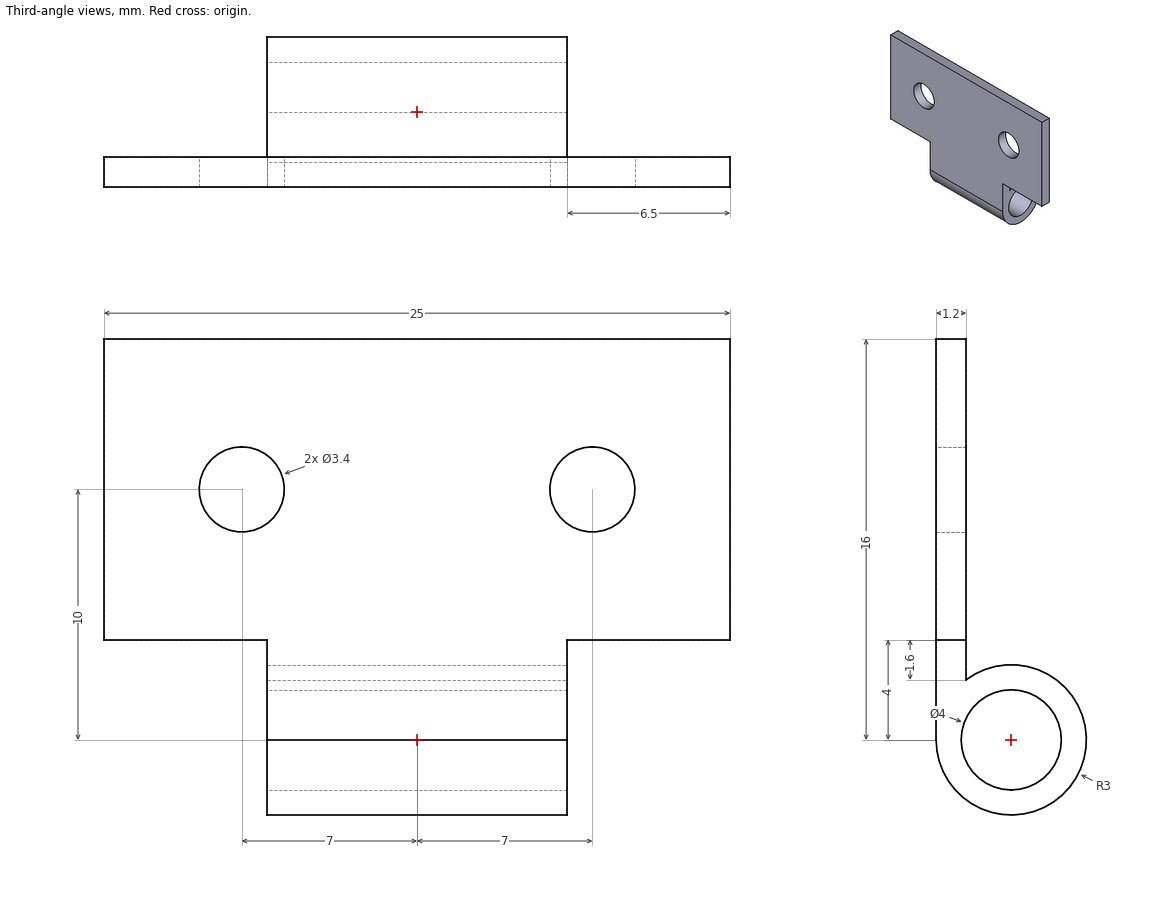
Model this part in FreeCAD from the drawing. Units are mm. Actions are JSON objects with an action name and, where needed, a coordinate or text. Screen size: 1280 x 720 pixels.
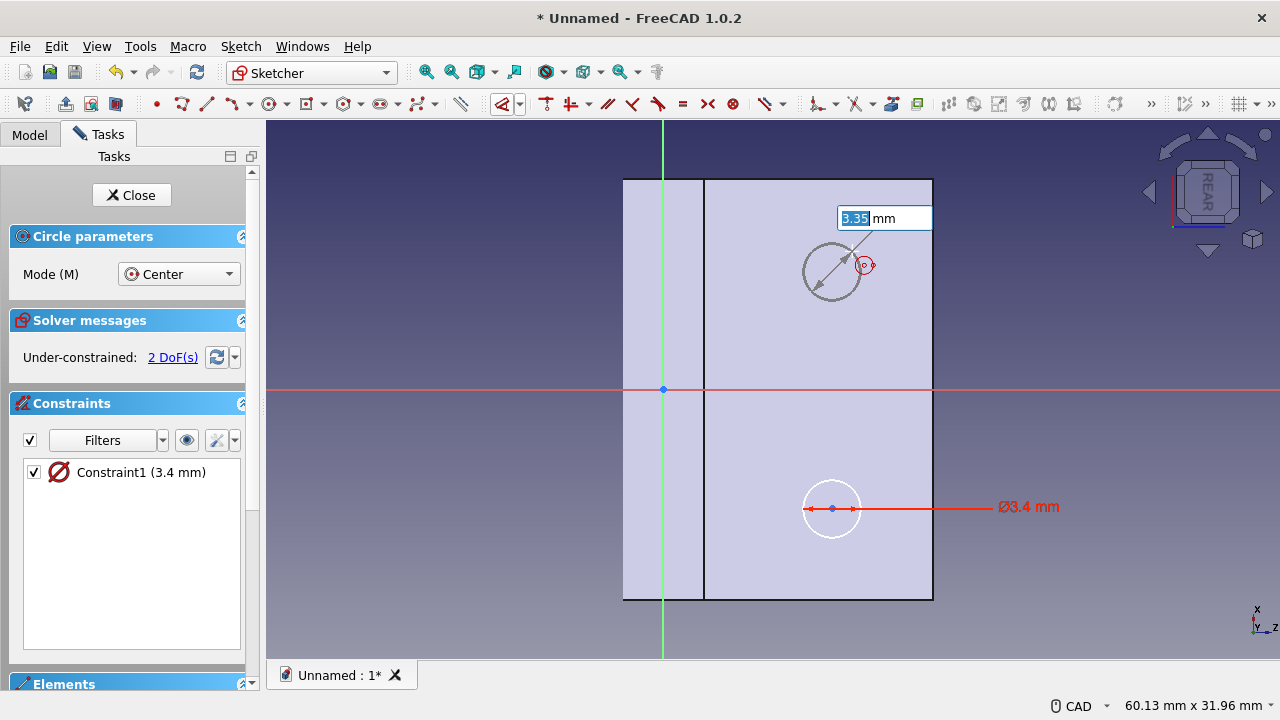
{"action": "type", "text": "3.4"}
{"action": "key", "text": "Return"}
{"action": "key", "text": "Escape"}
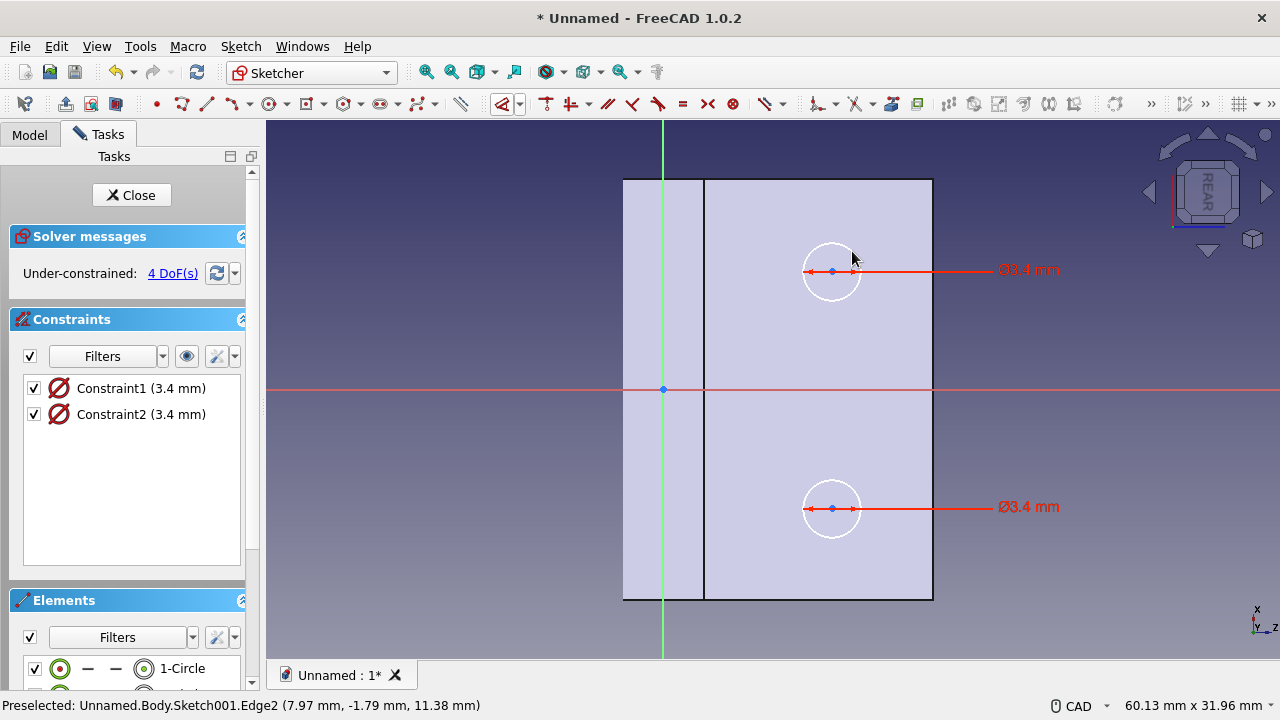
{"action": "left_click", "coordinate": [832, 509]}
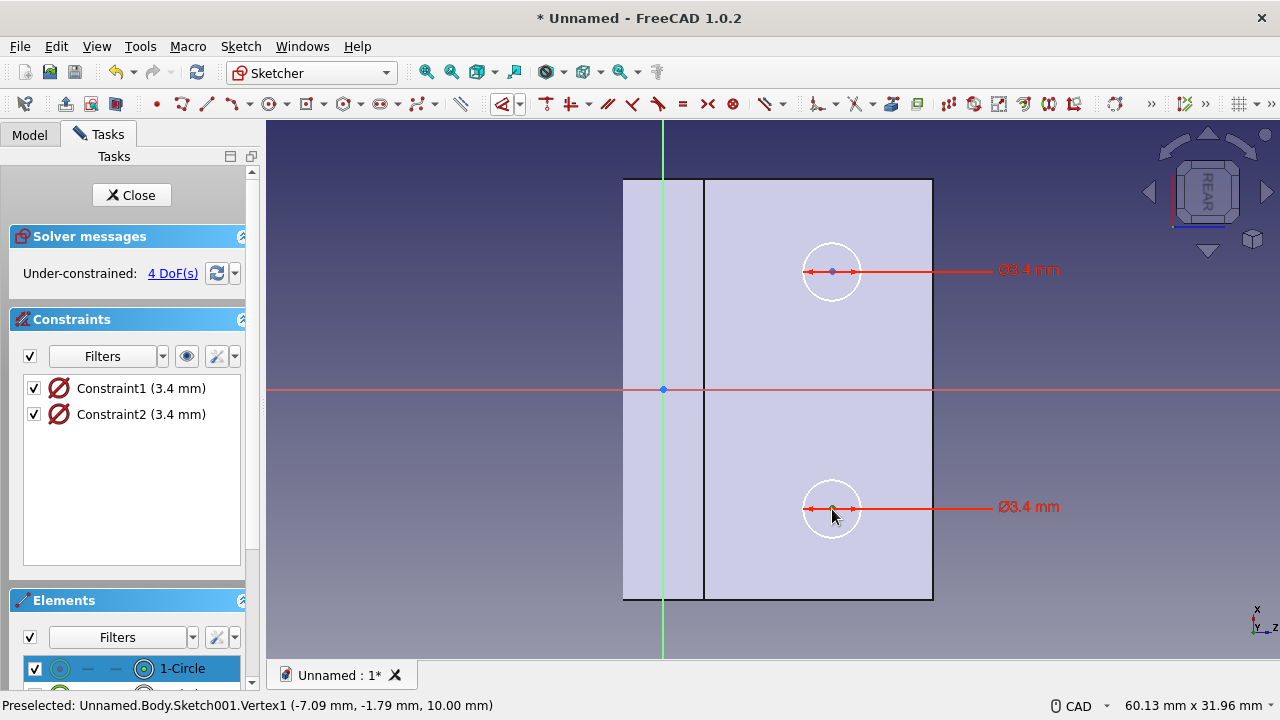
{"action": "left_click", "coordinate": [832, 272]}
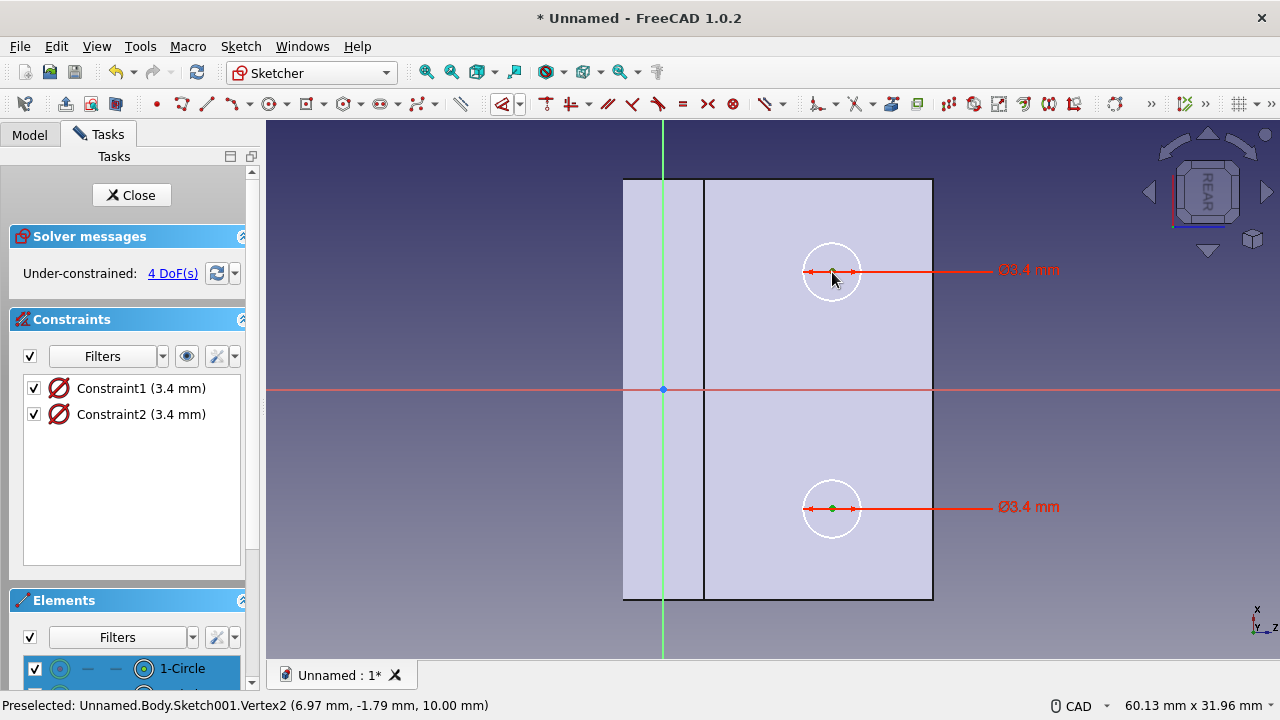
{"action": "key", "text": "v"}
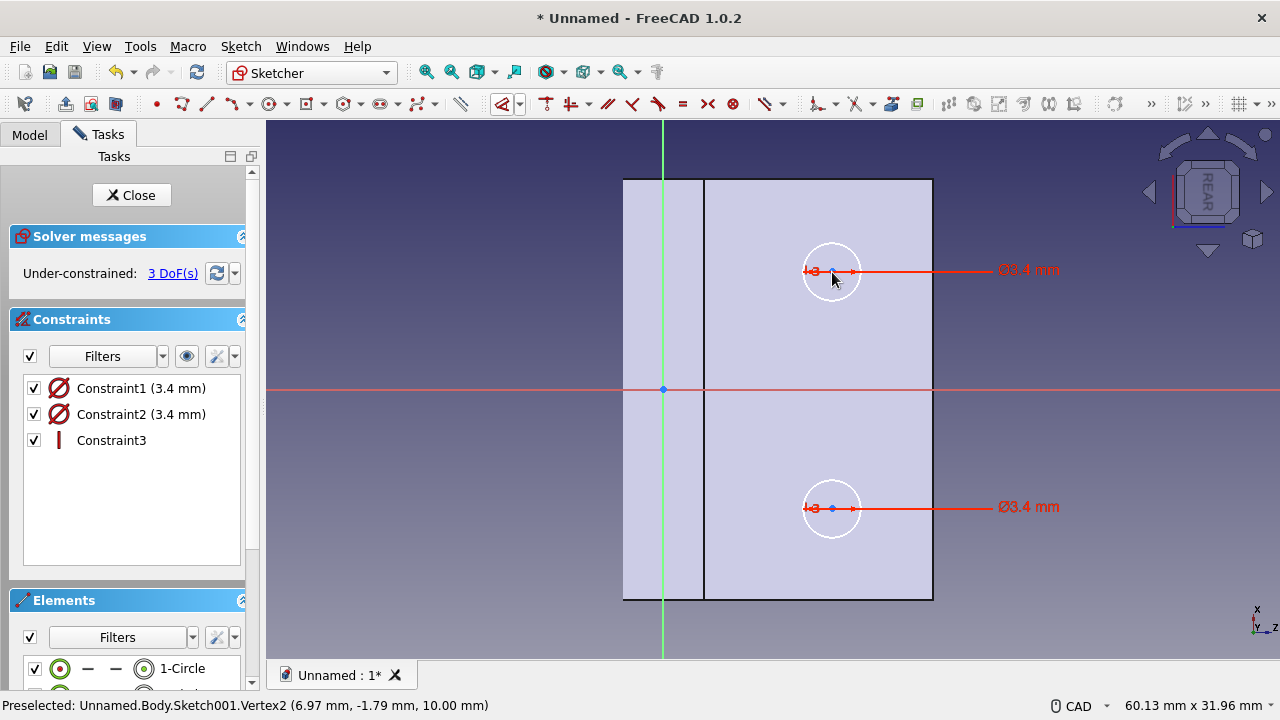
{"action": "left_click", "coordinate": [832, 509]}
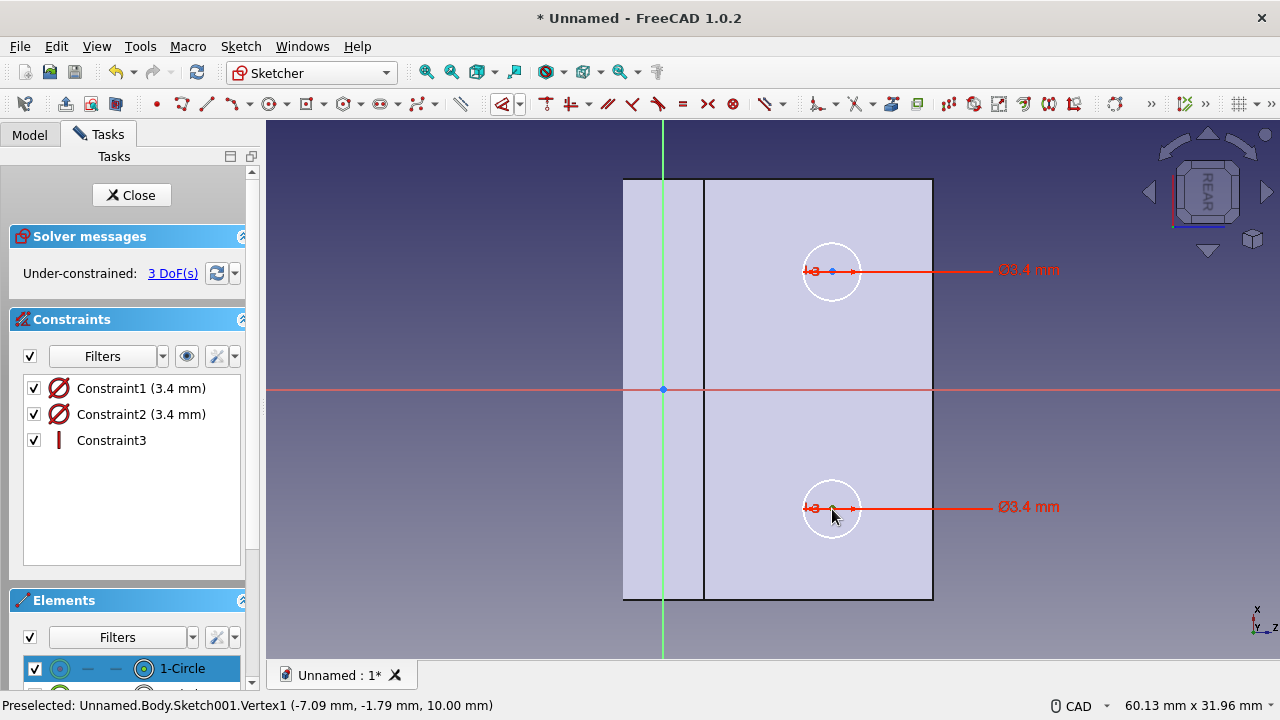
{"action": "left_click", "coordinate": [520, 104]}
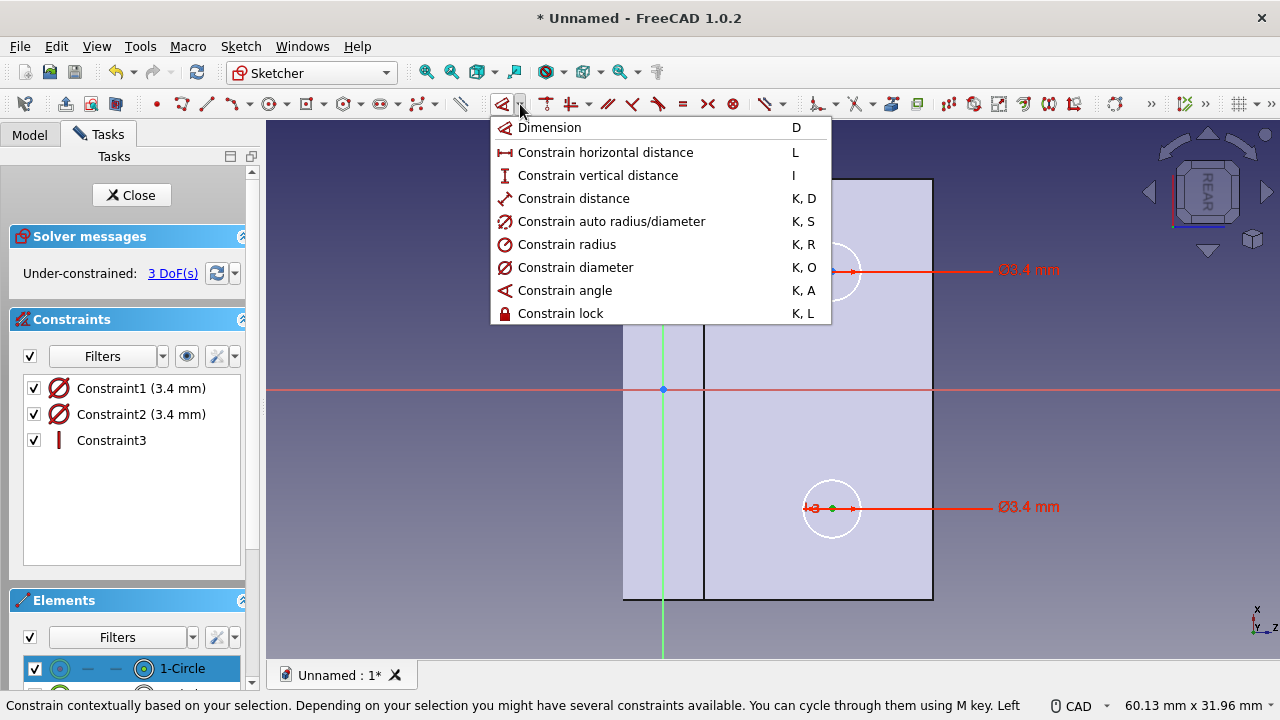
{"action": "left_click", "coordinate": [661, 176]}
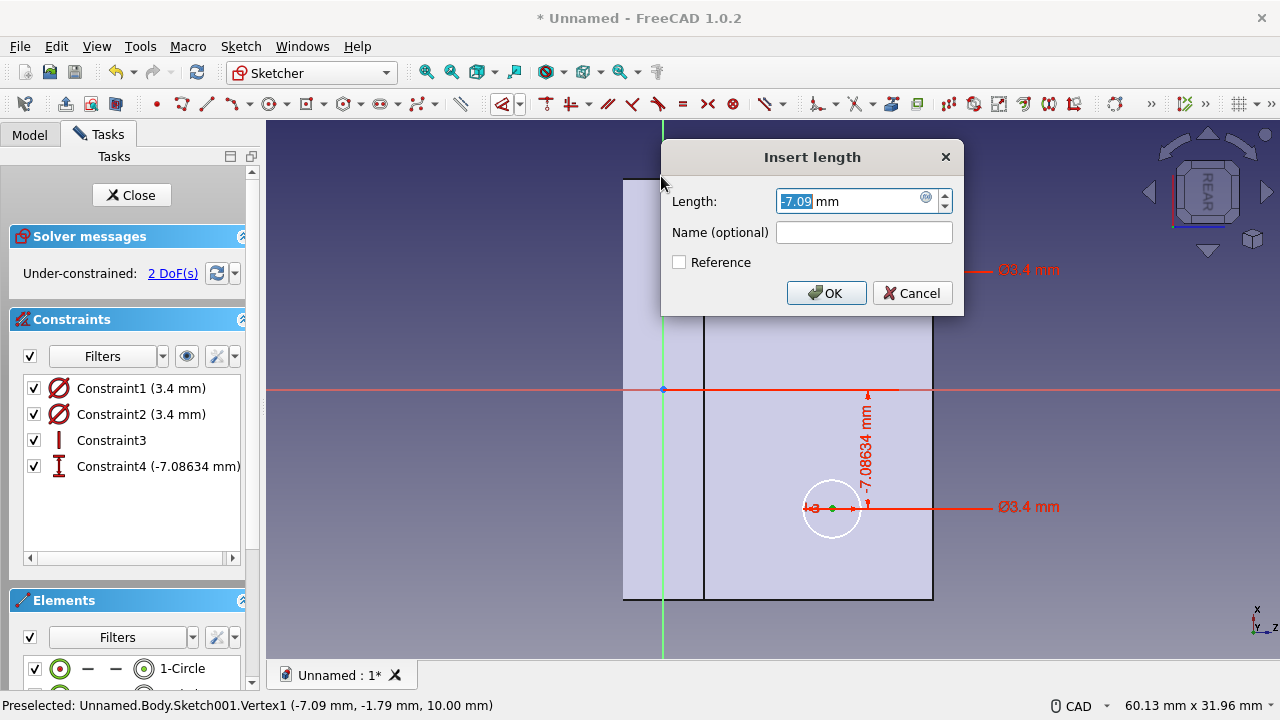
{"action": "type", "text": "-7"}
{"action": "key", "text": "Return"}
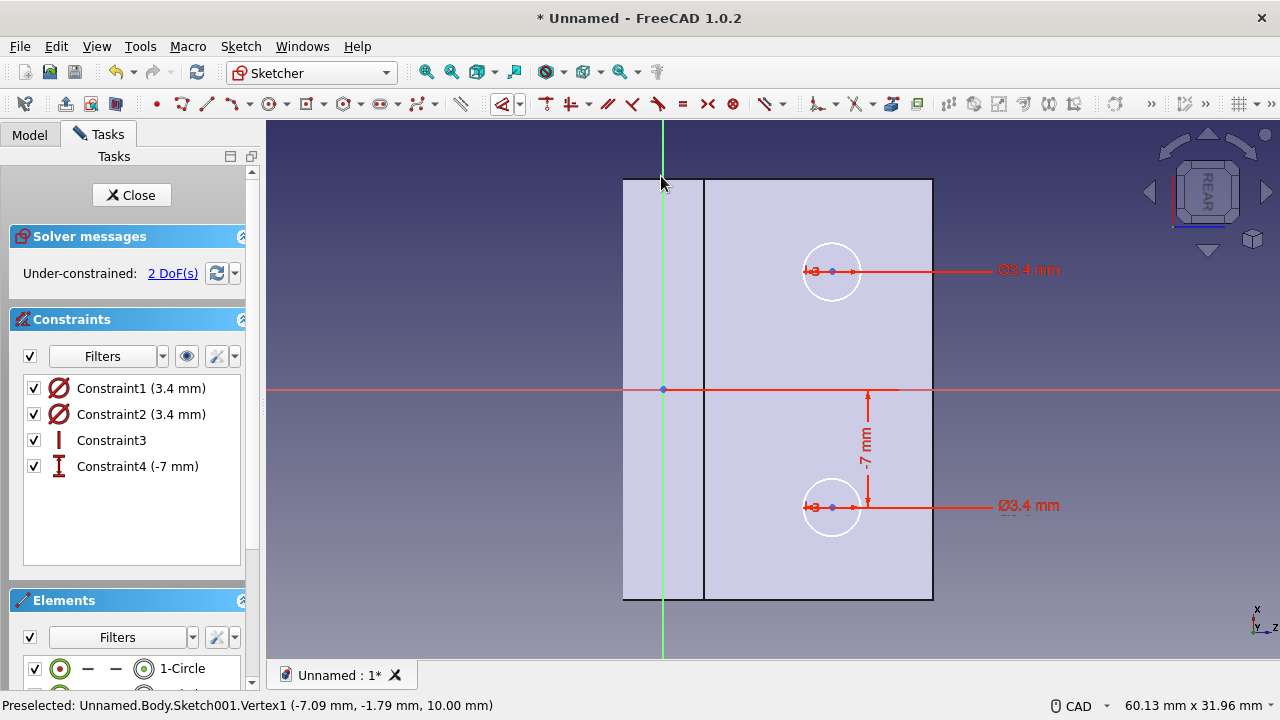
{"action": "left_click", "coordinate": [832, 272]}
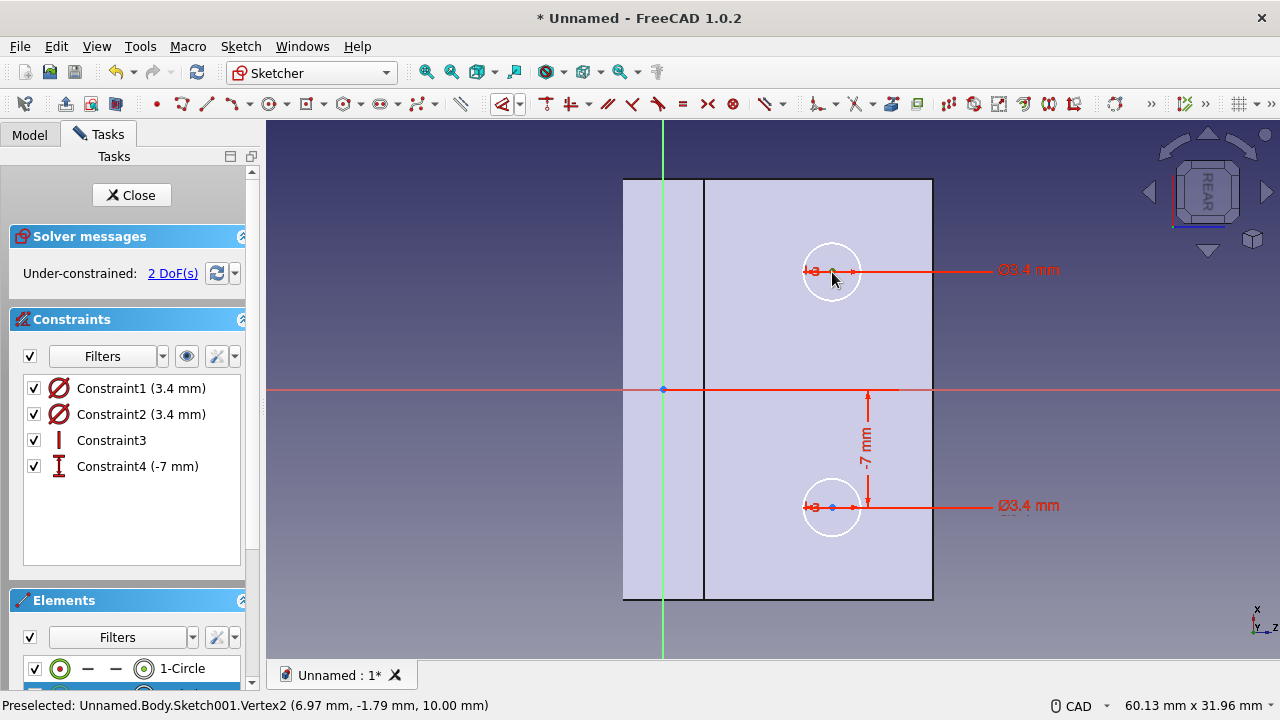
{"action": "left_click", "coordinate": [520, 104]}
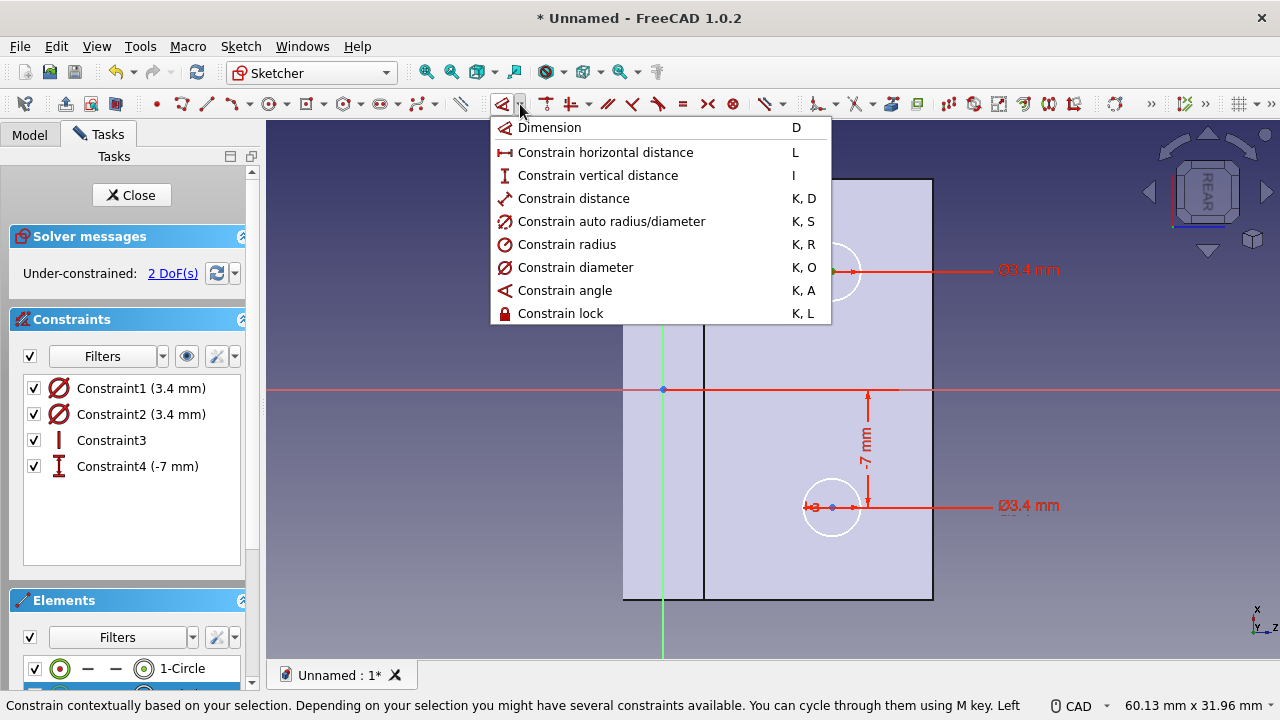
{"action": "left_click", "coordinate": [661, 176]}